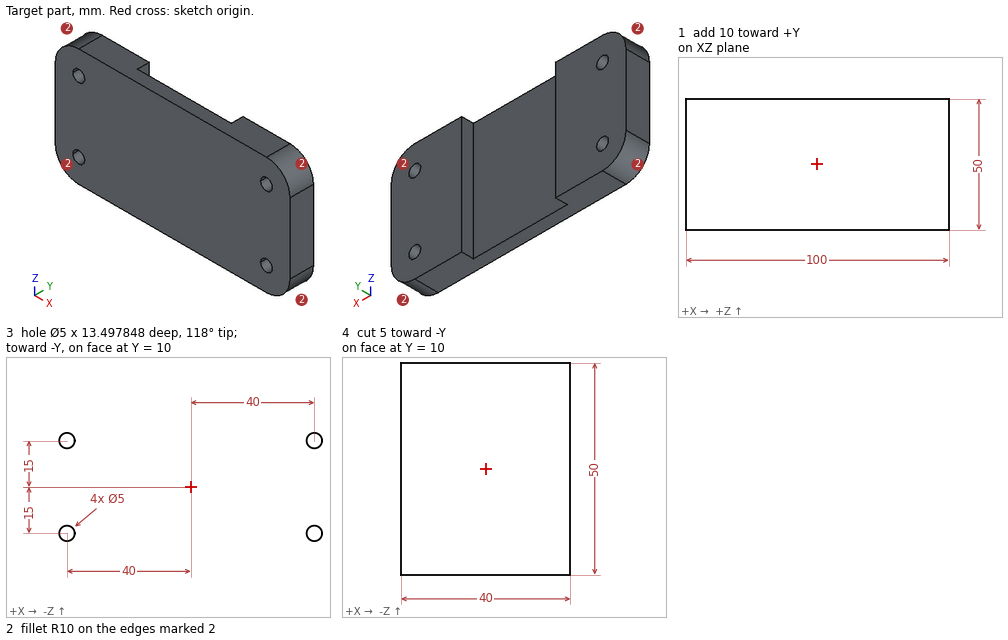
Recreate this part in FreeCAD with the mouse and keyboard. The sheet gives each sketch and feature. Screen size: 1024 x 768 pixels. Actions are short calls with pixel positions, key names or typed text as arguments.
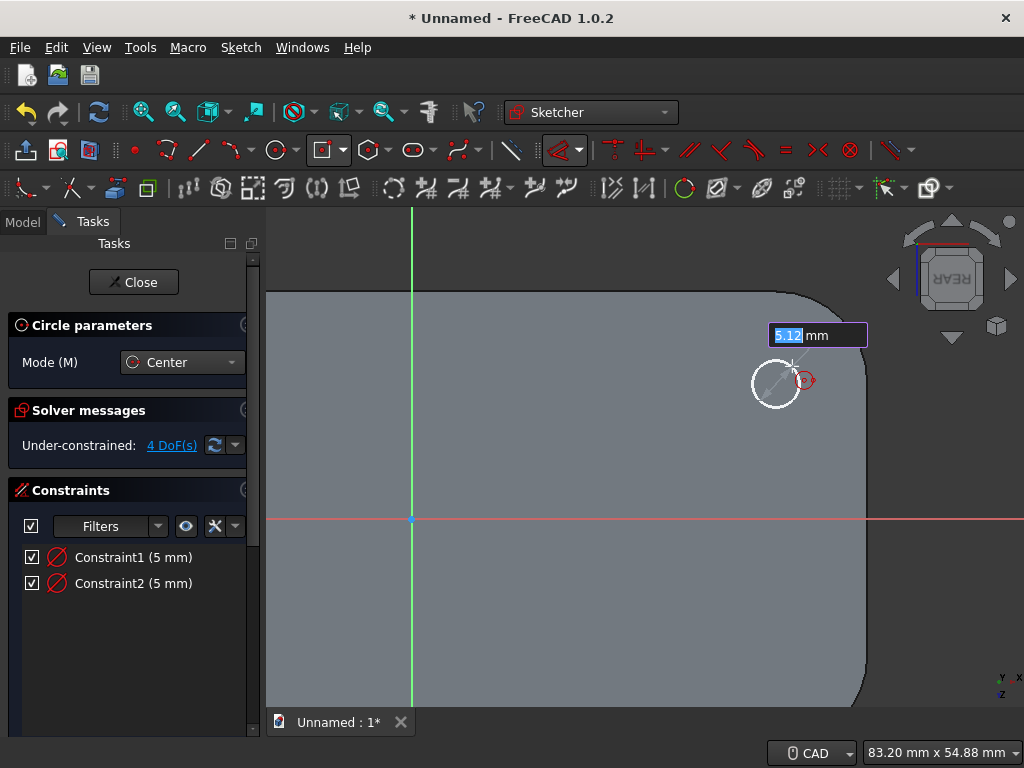
text(5)
key(Return)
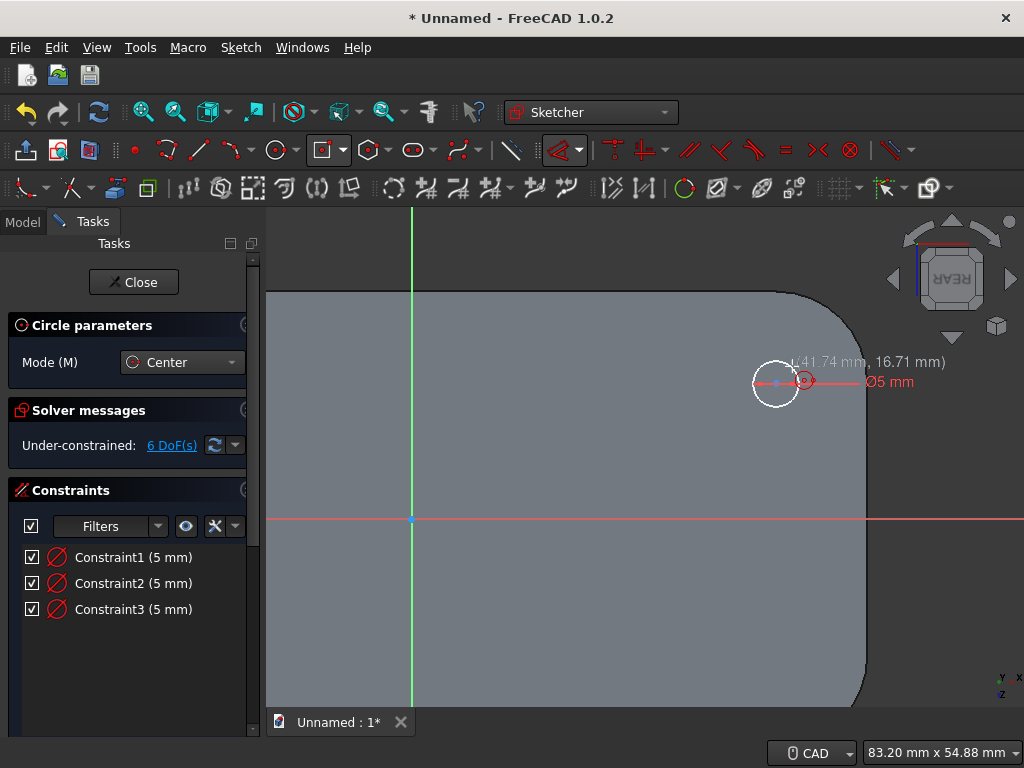
click(776, 656)
move(792, 640)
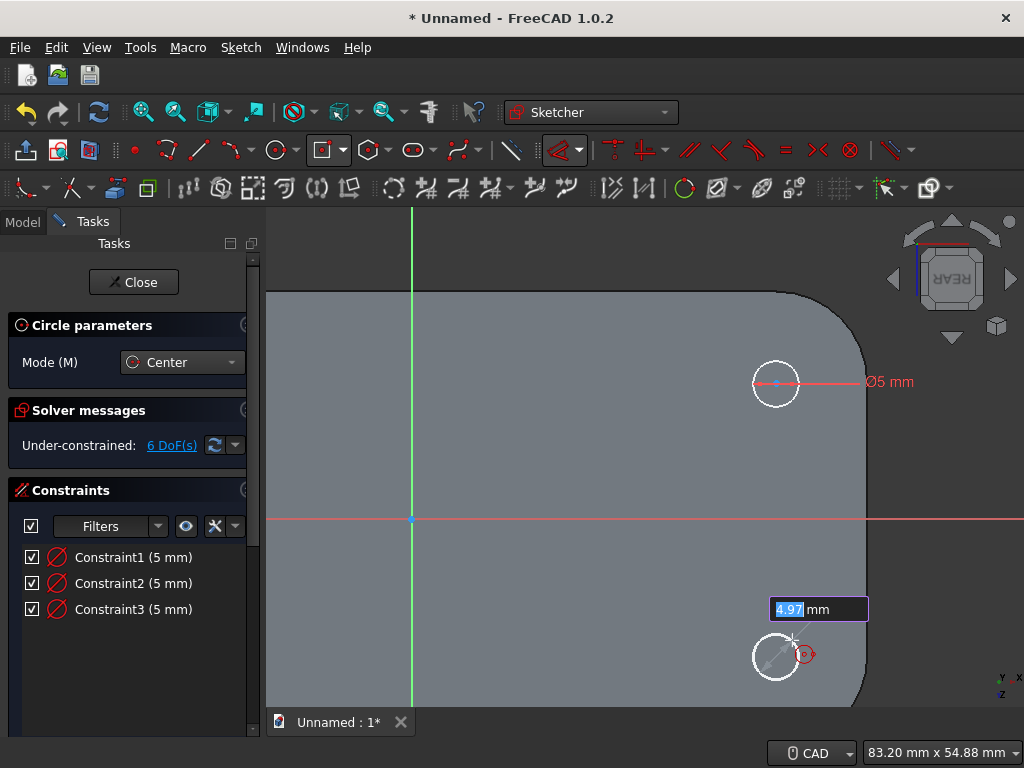
text(5)
key(Return)
key(Escape)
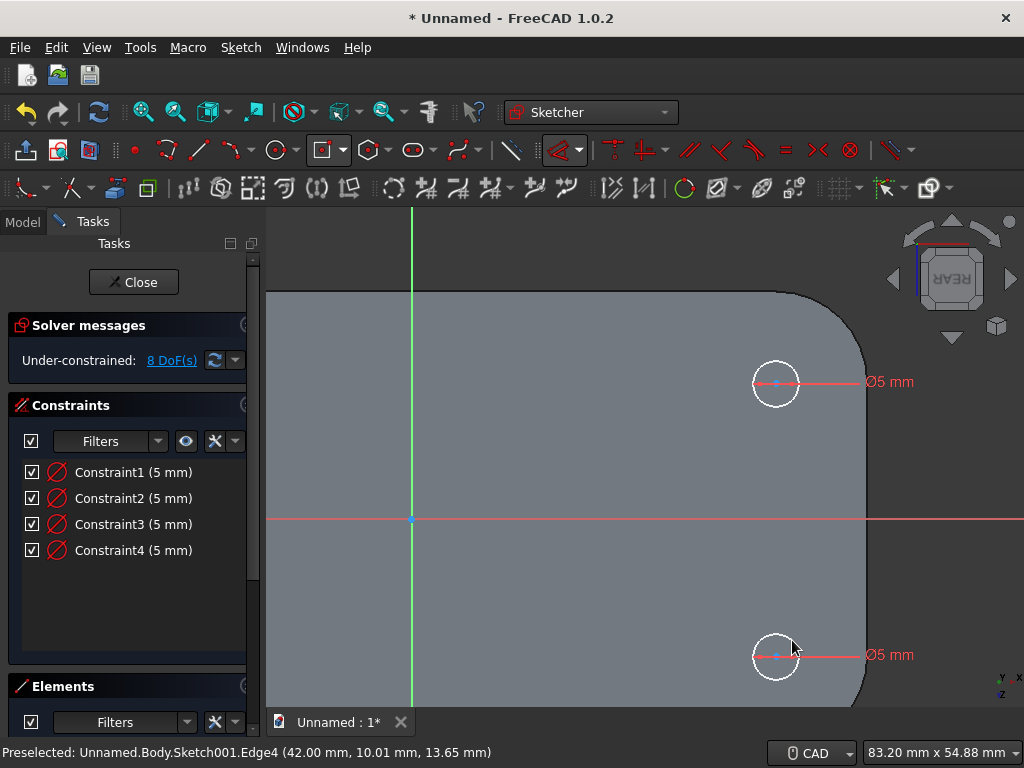
scroll(777, 381, down, 3)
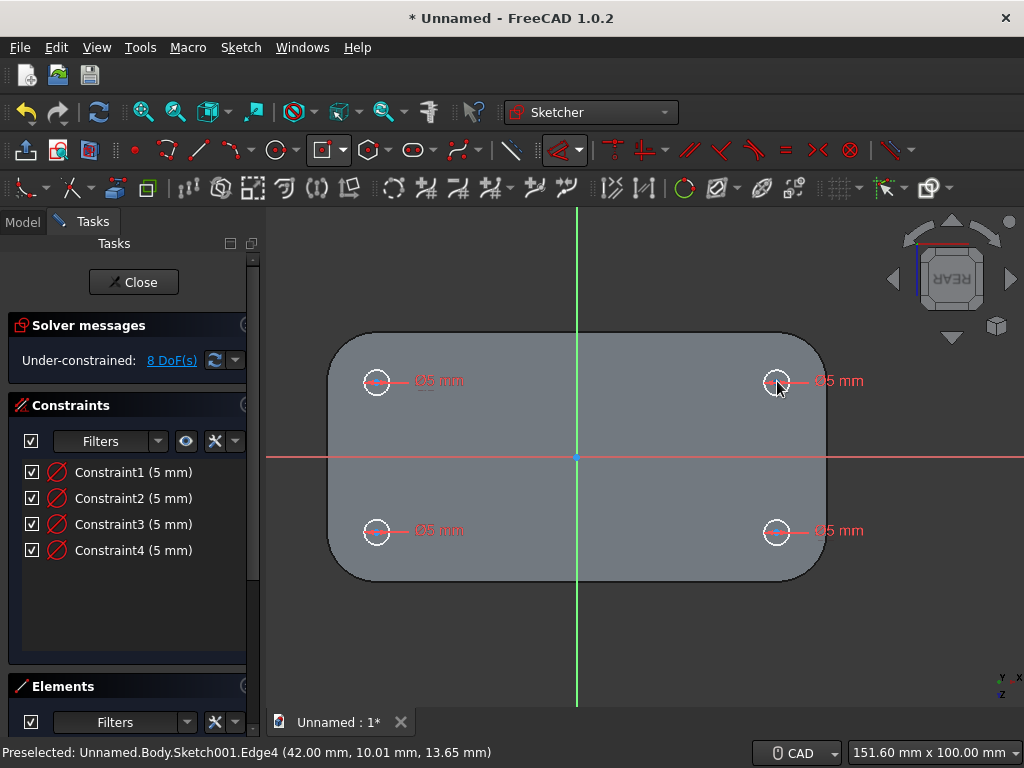
click(377, 532)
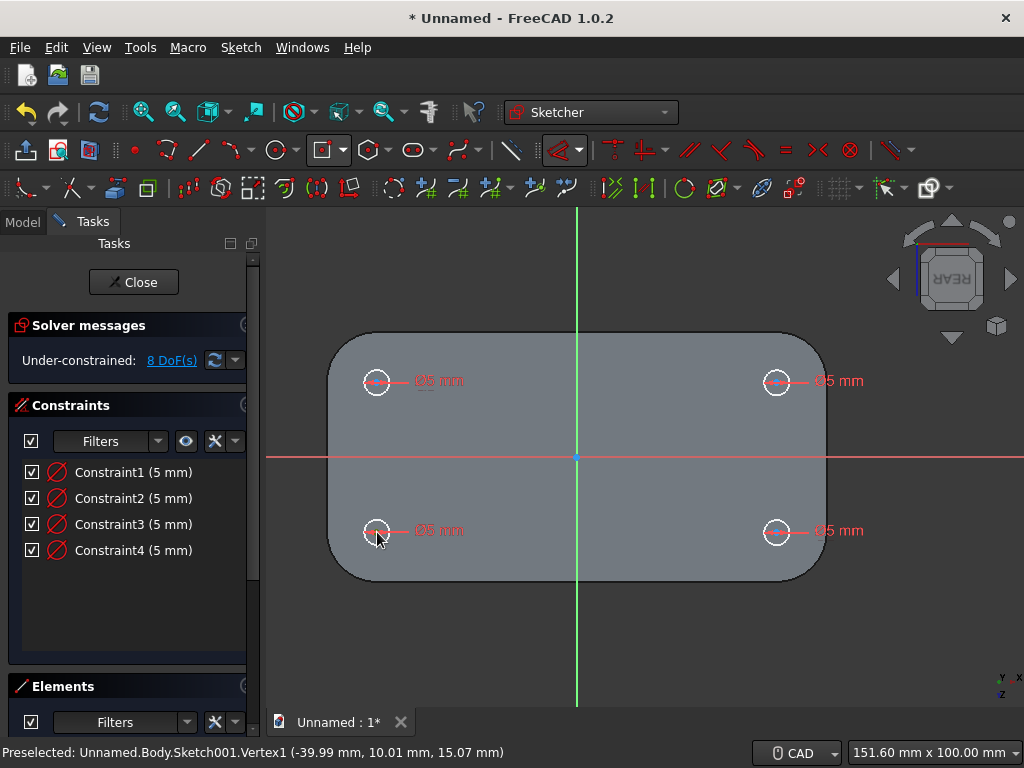
click(377, 383)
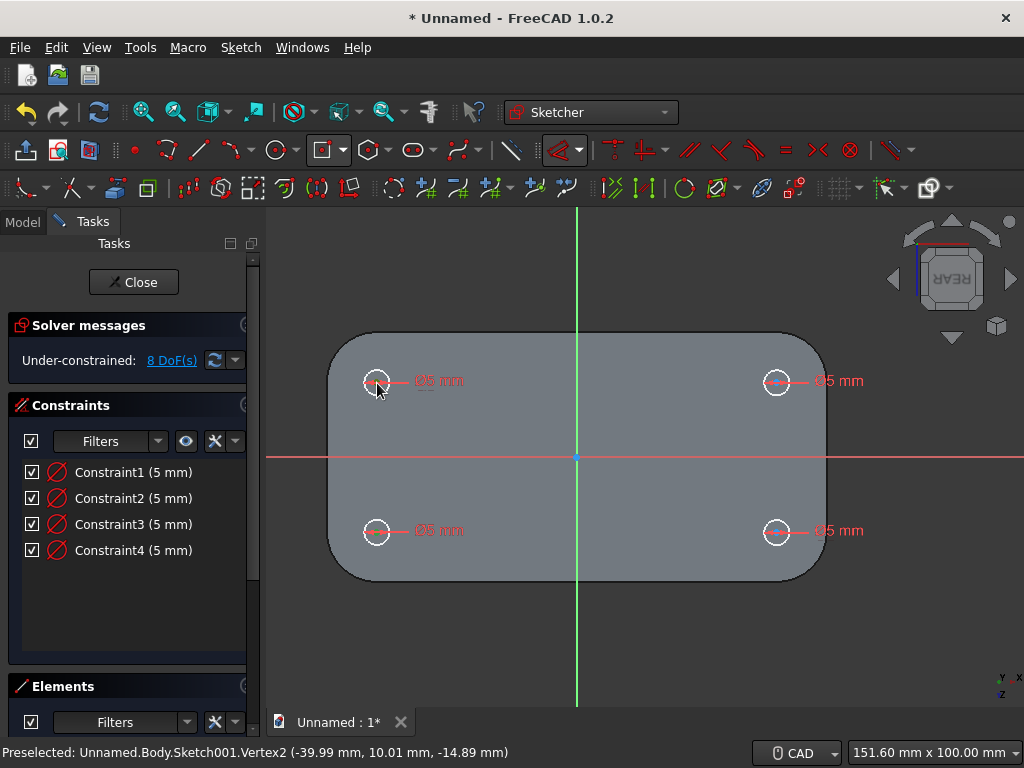
click(668, 150)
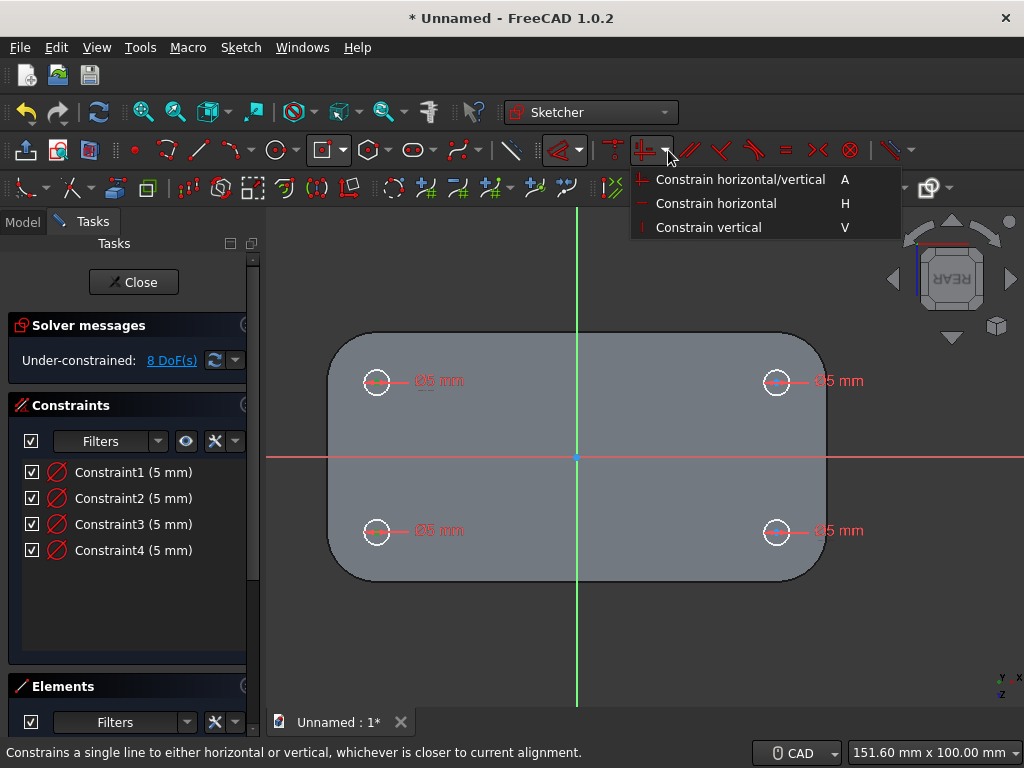
click(766, 227)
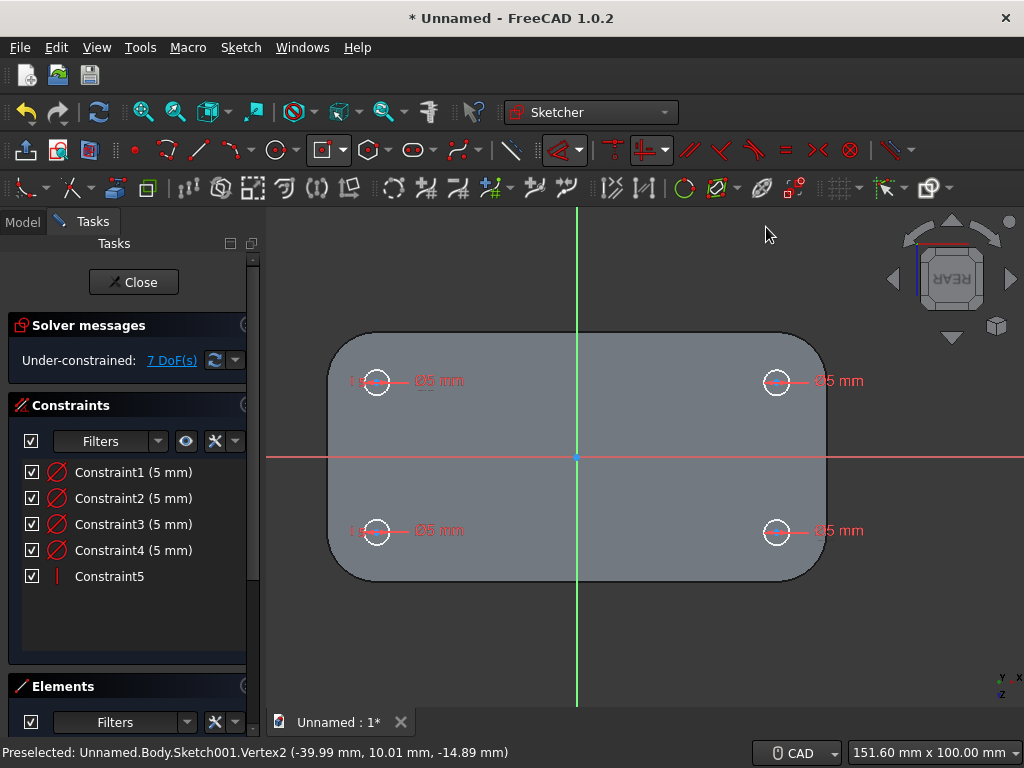
click(377, 383)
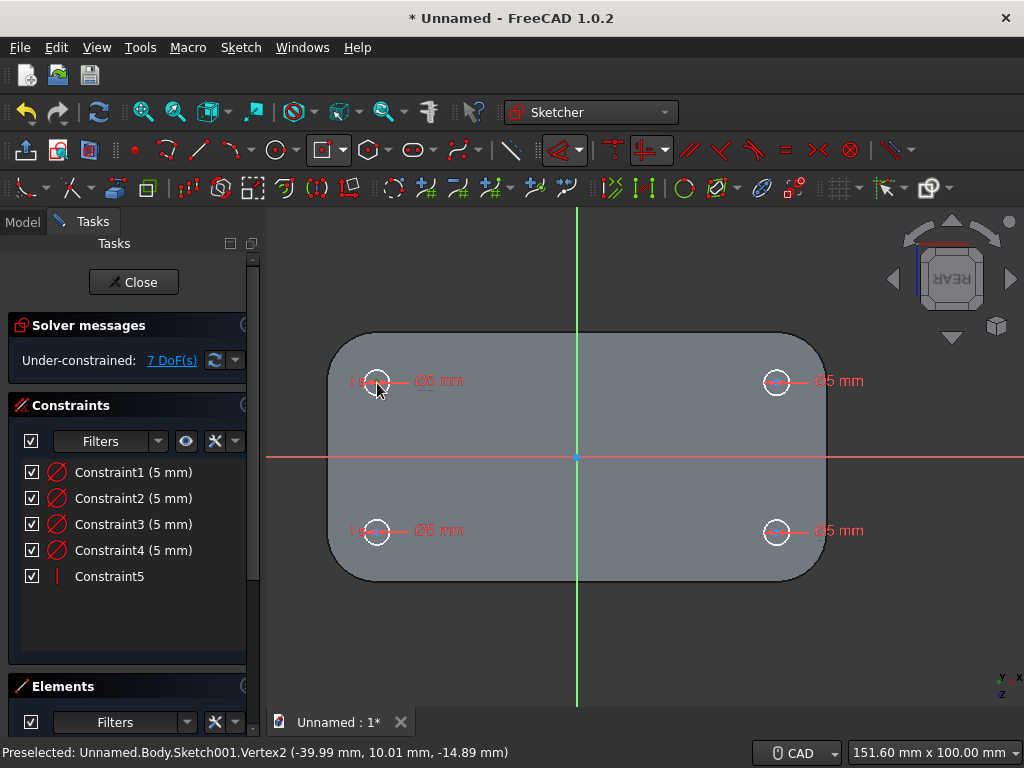
click(777, 383)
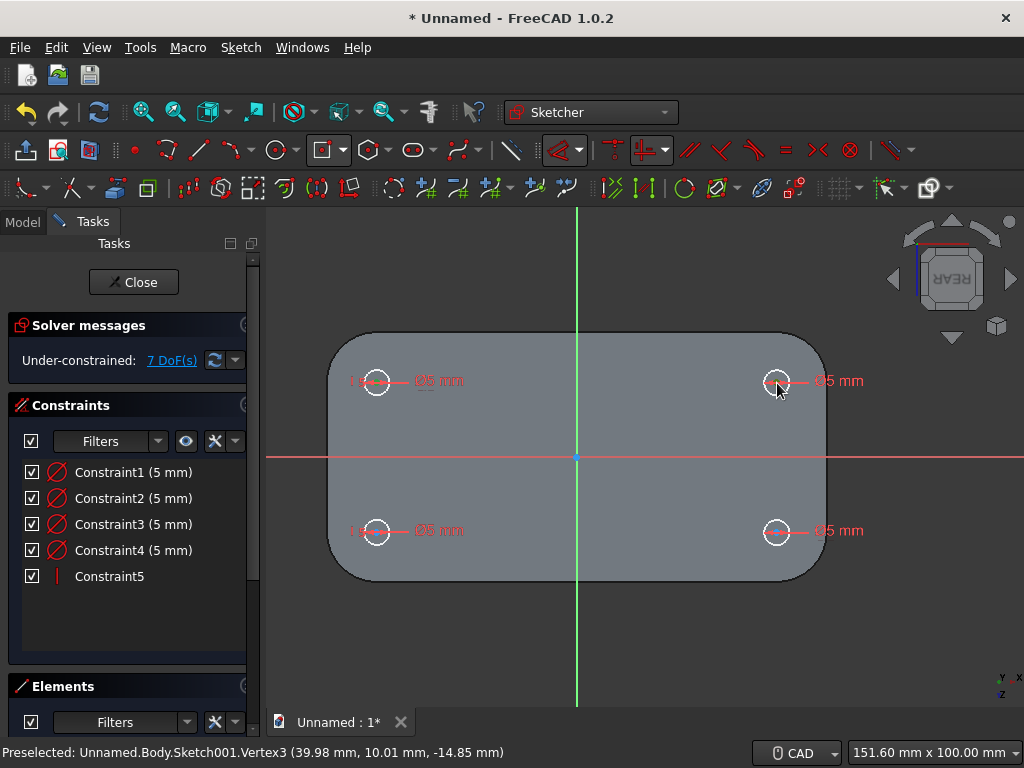
key(h)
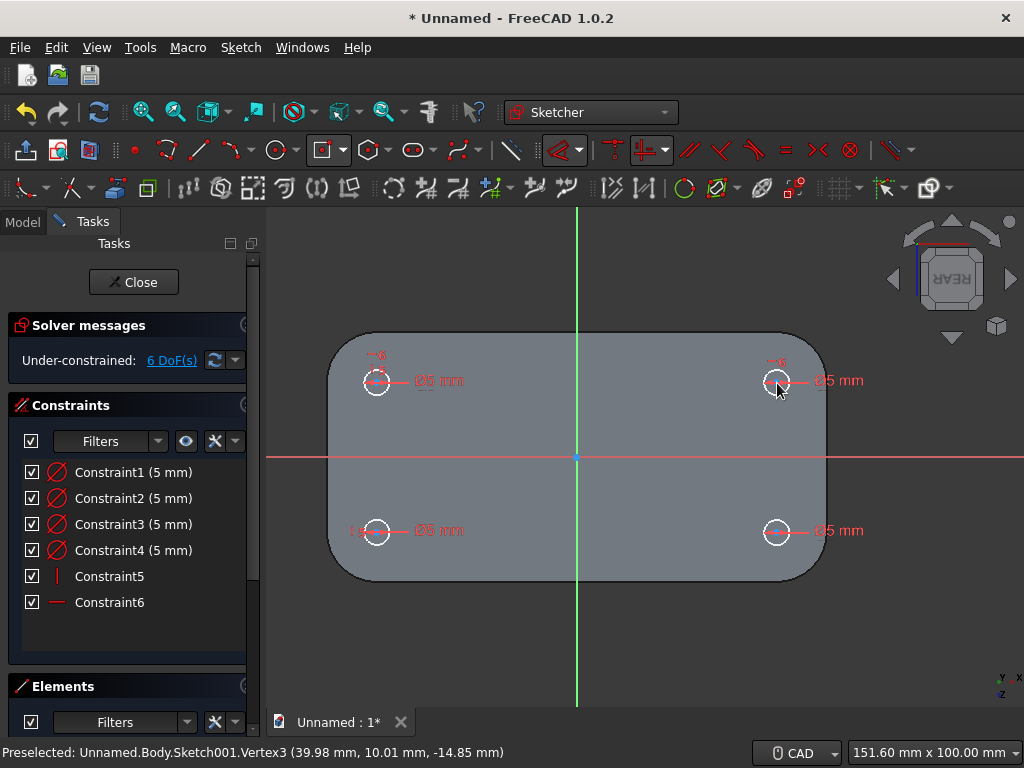
click(777, 383)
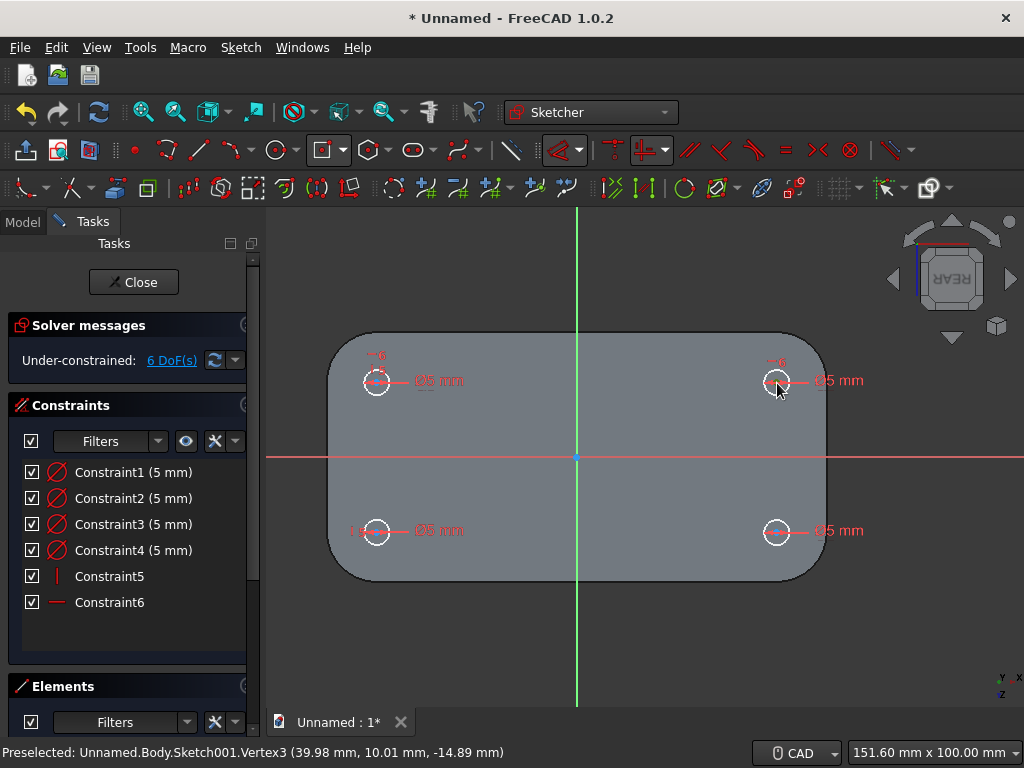
click(777, 533)